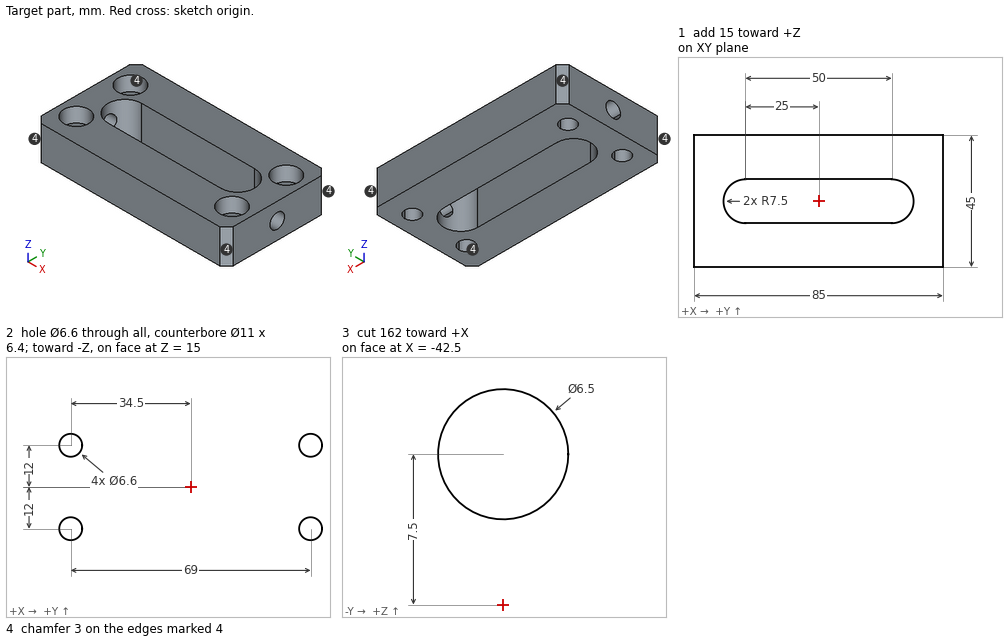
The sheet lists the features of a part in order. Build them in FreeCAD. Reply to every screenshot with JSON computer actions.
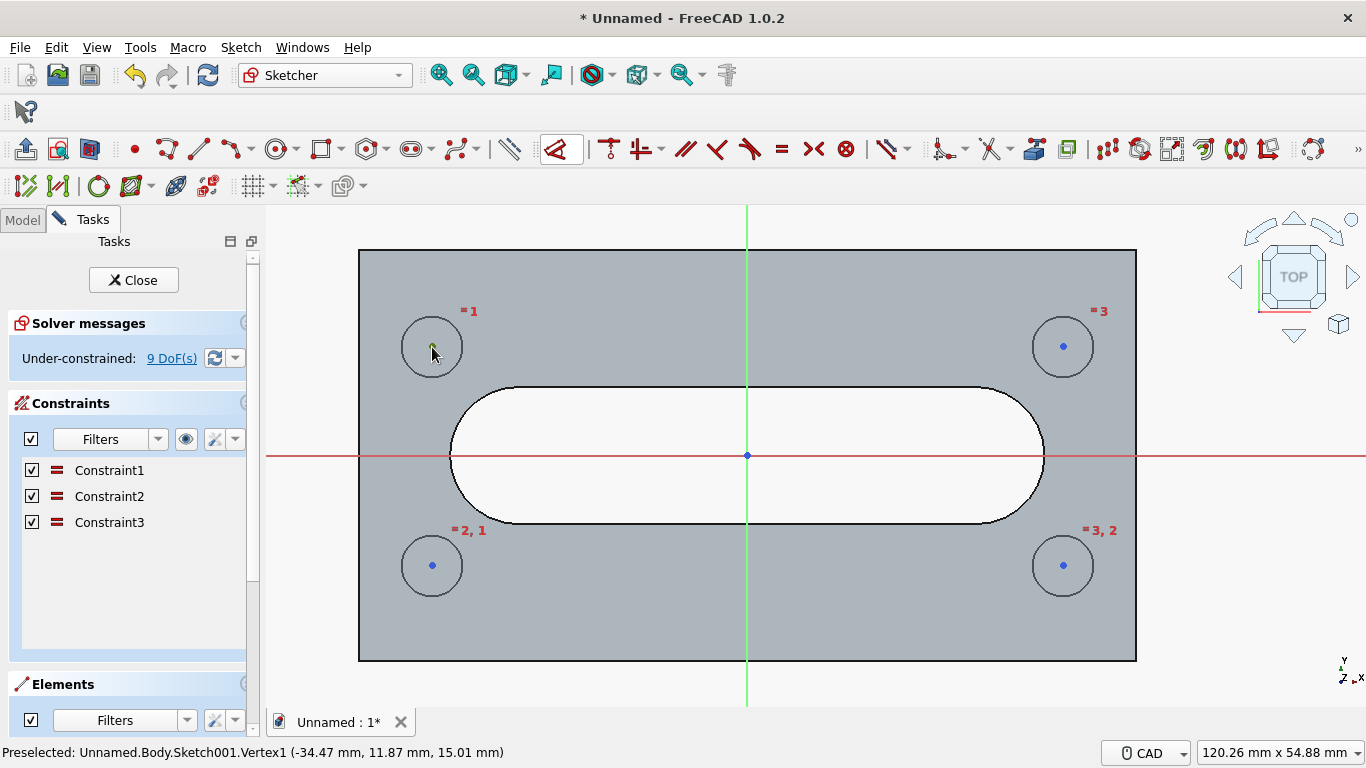
{"action": "left_click", "coordinate": [432, 566]}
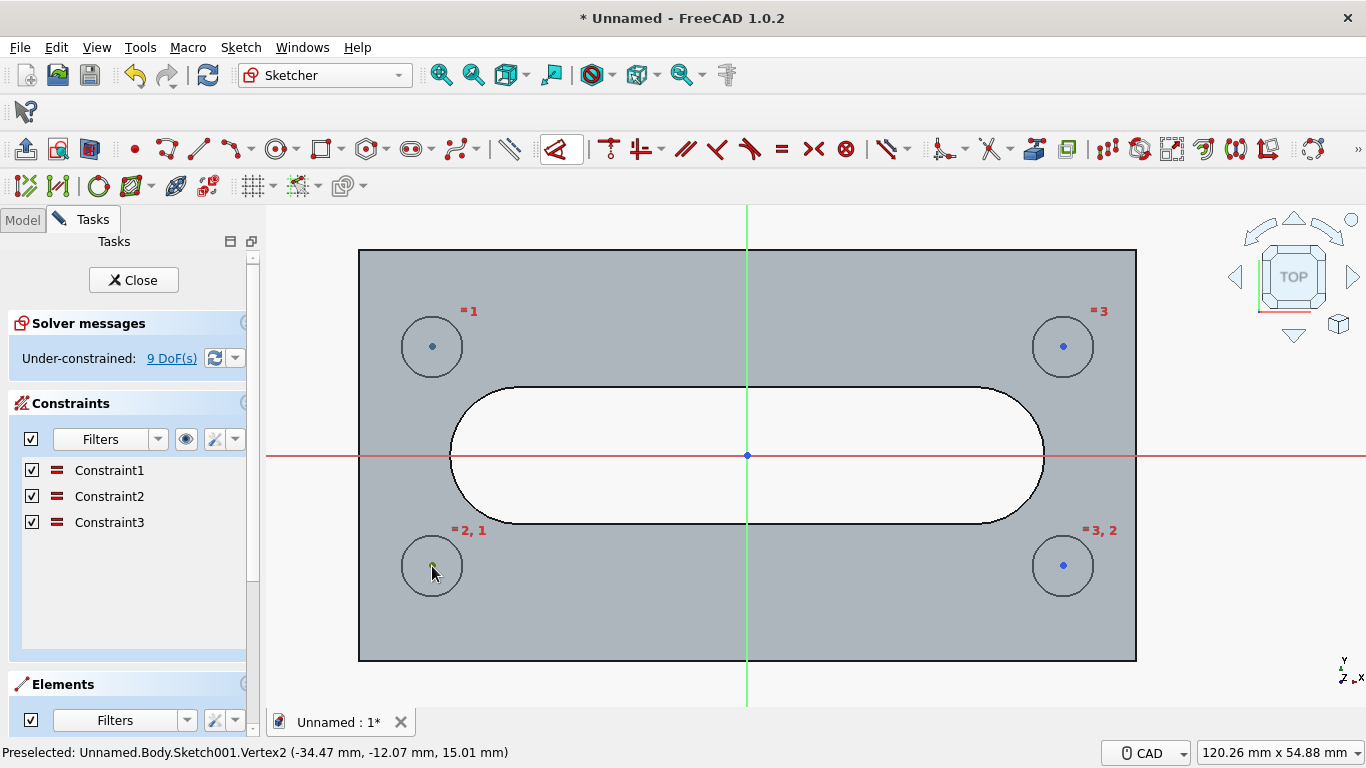
{"action": "left_click", "coordinate": [664, 150]}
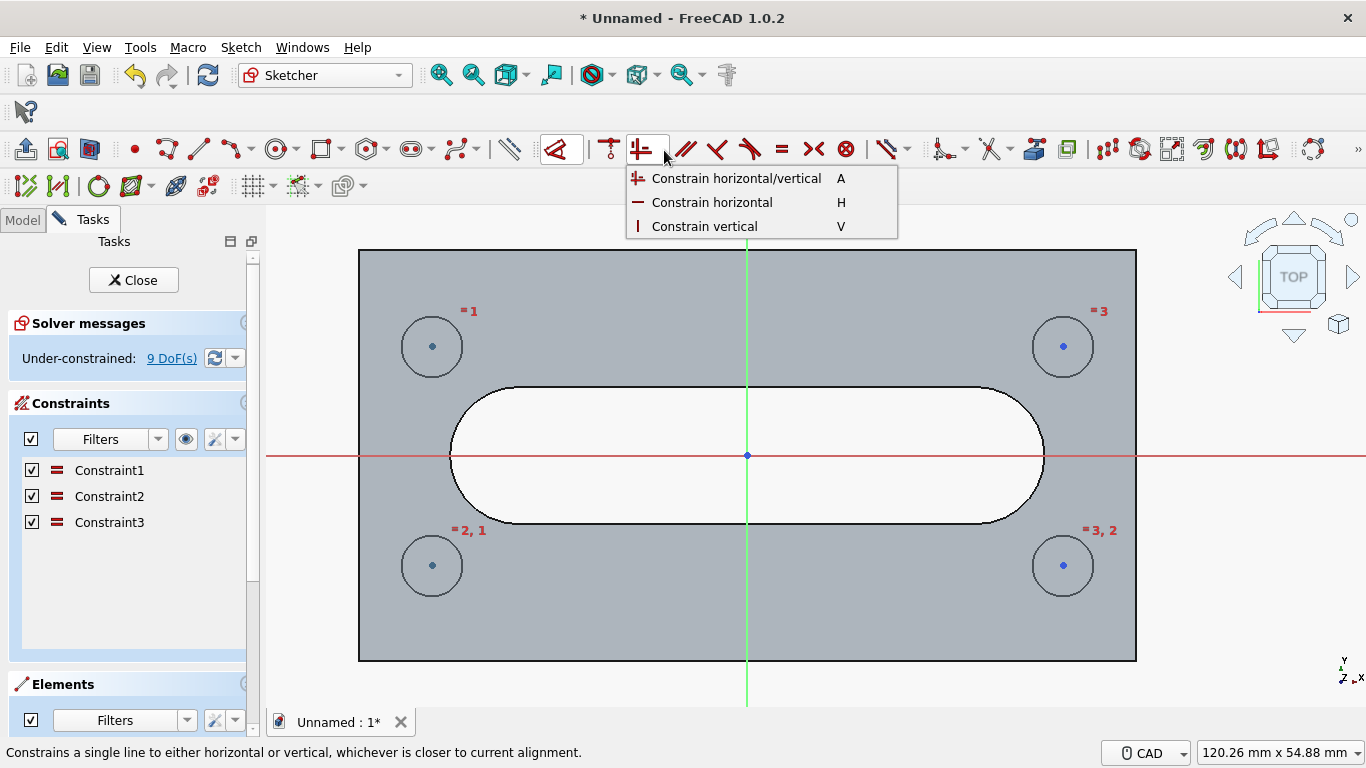
{"action": "left_click", "coordinate": [762, 226]}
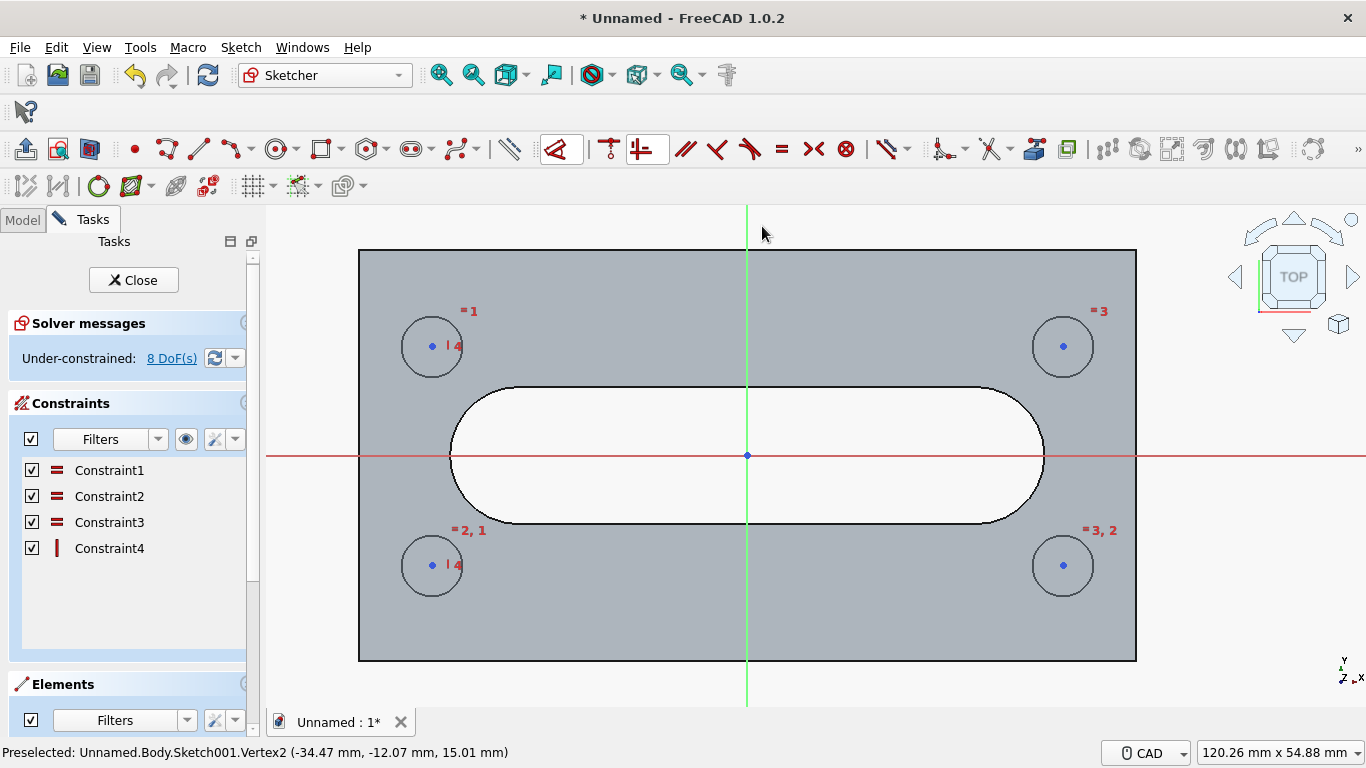
{"action": "left_click", "coordinate": [432, 566]}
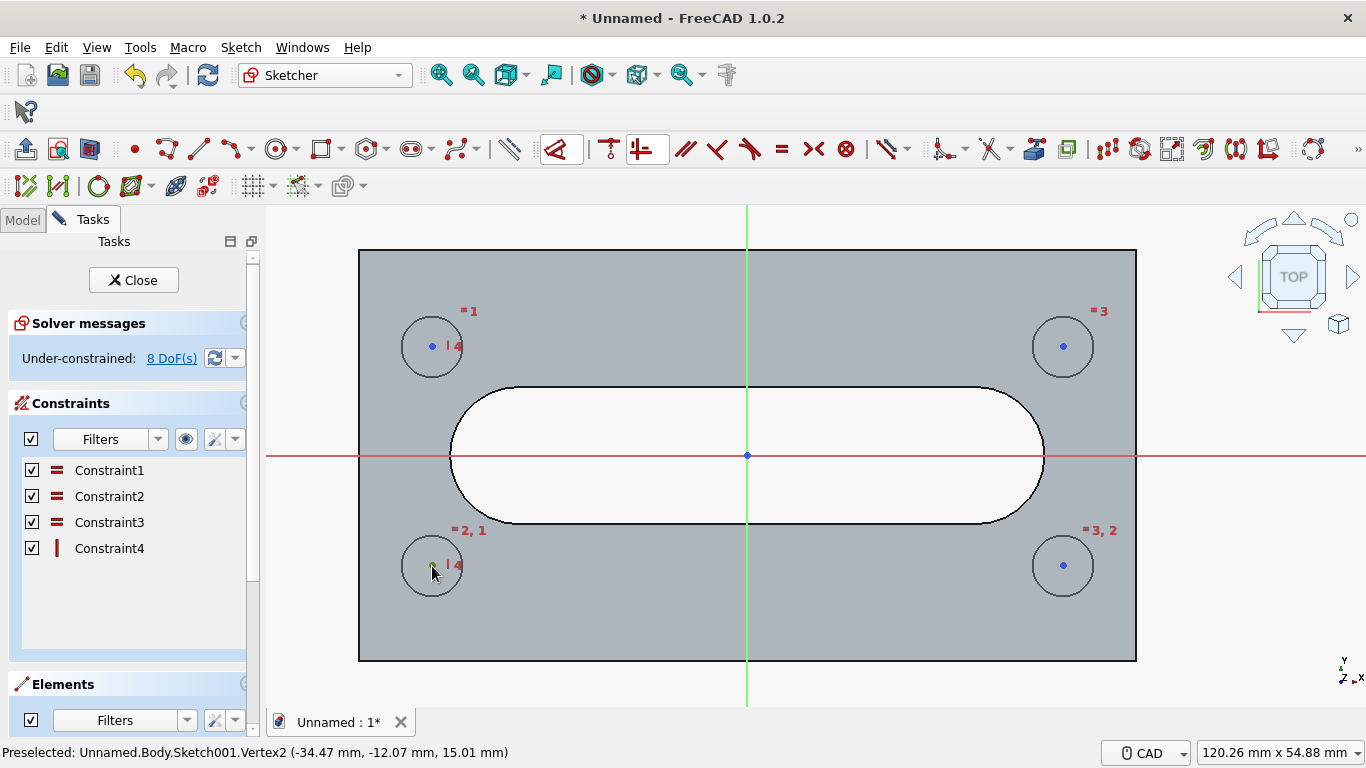
{"action": "left_click", "coordinate": [1063, 566]}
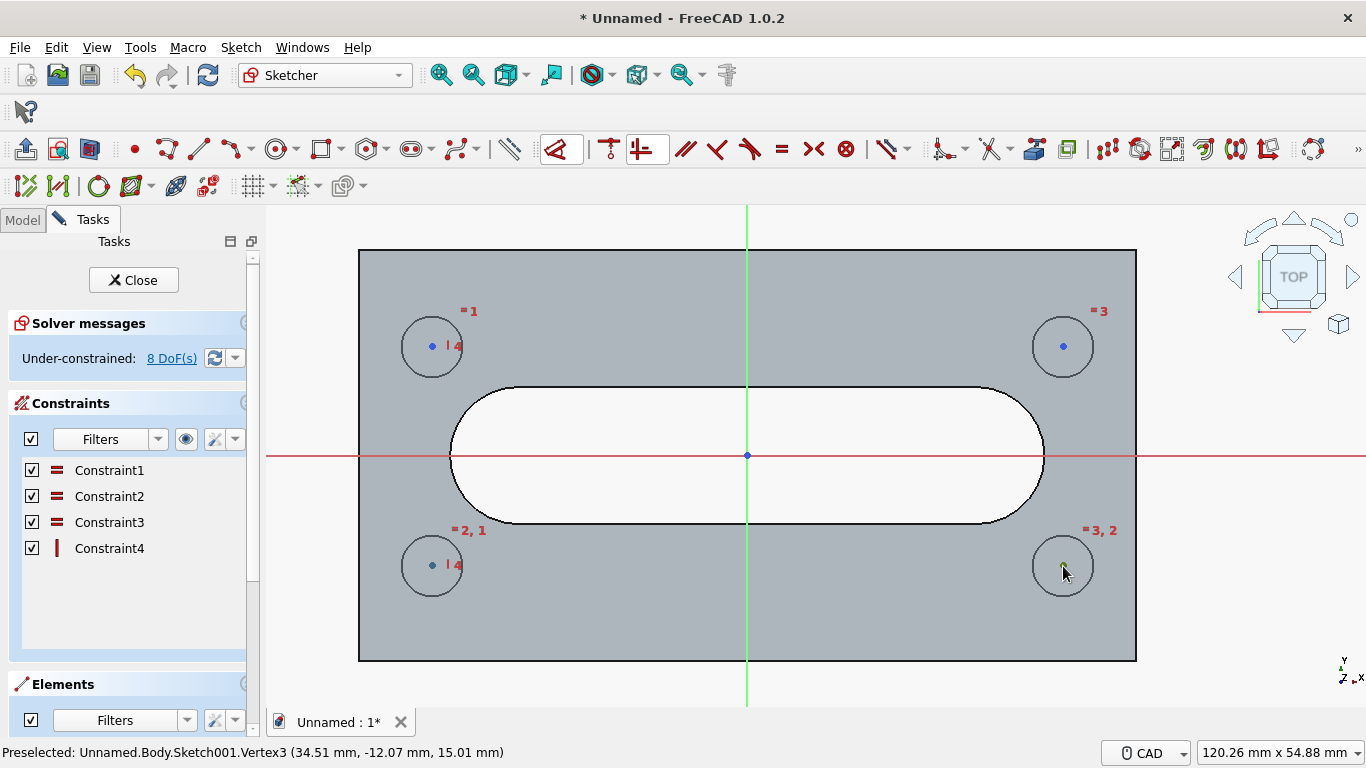
{"action": "left_click", "coordinate": [664, 150]}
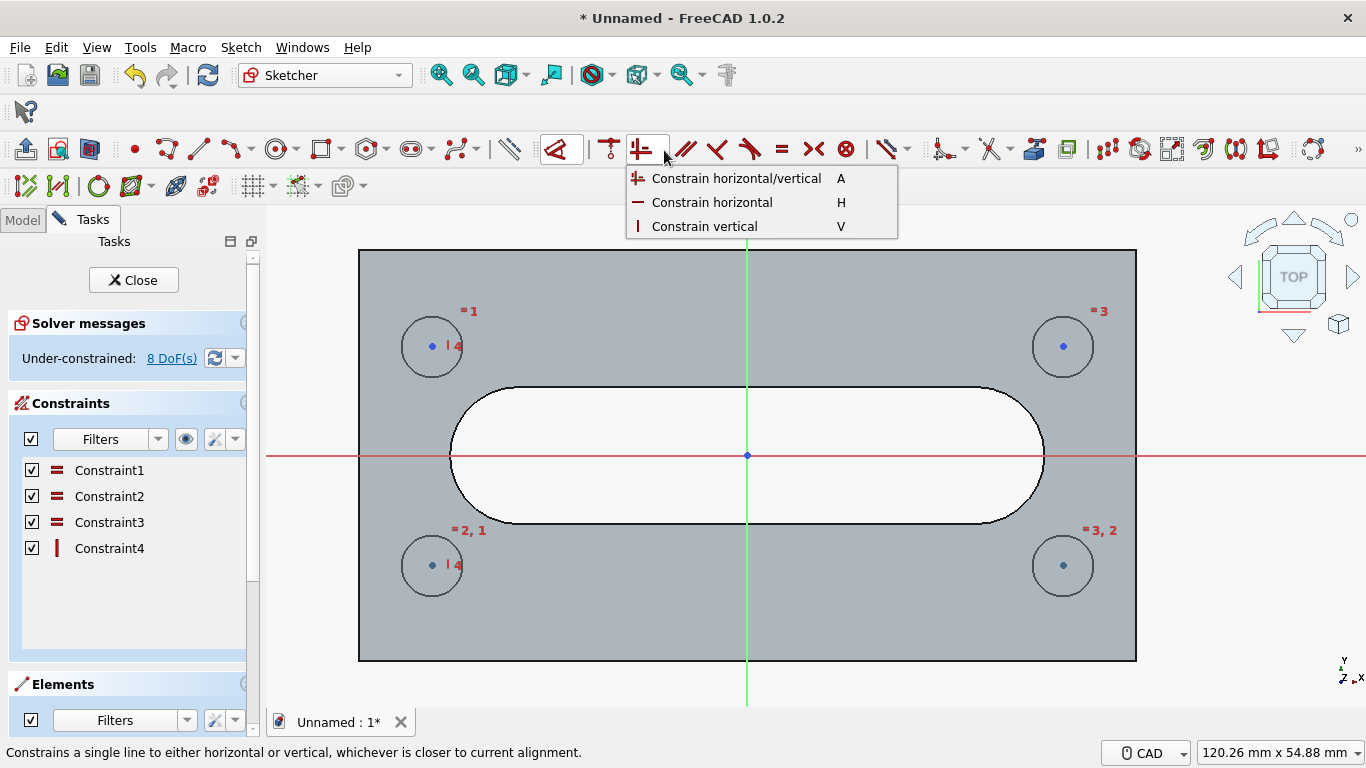
{"action": "left_click", "coordinate": [762, 202]}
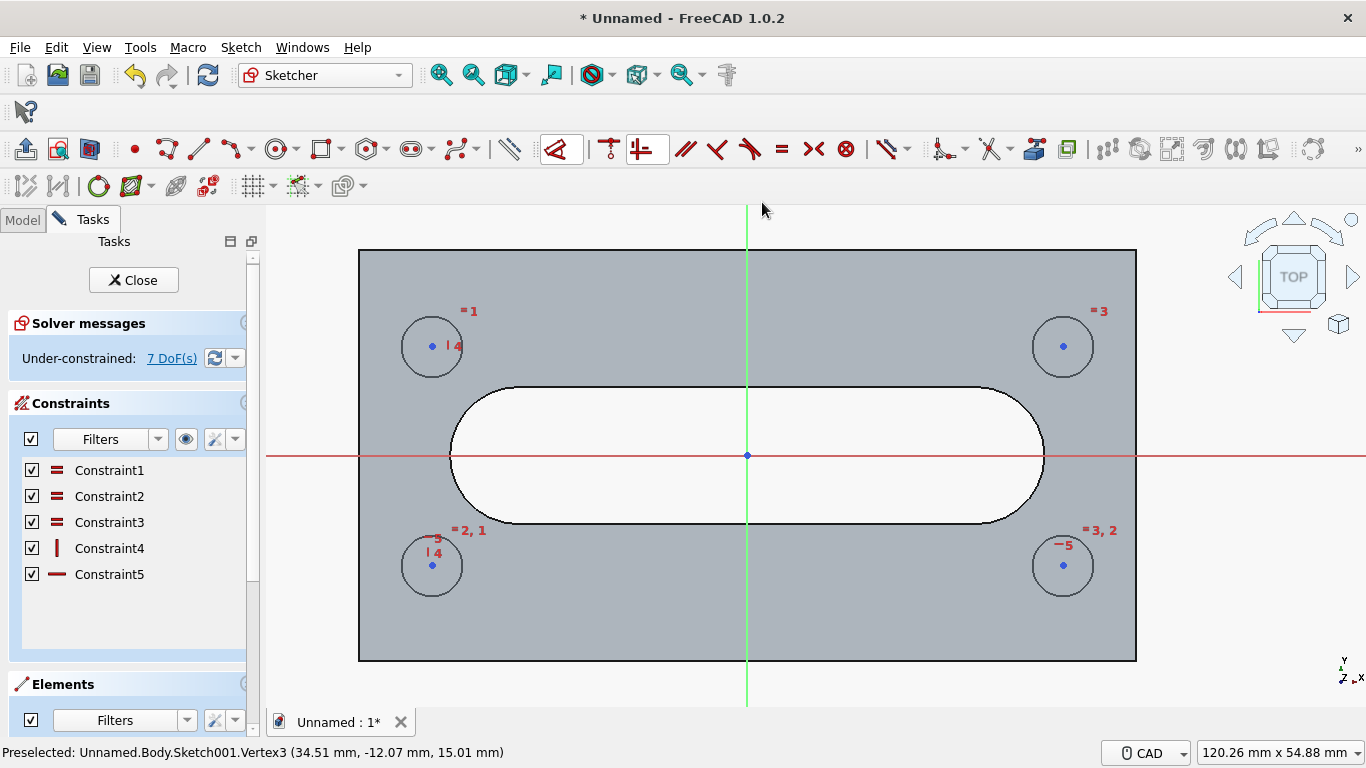
{"action": "left_click", "coordinate": [1063, 566]}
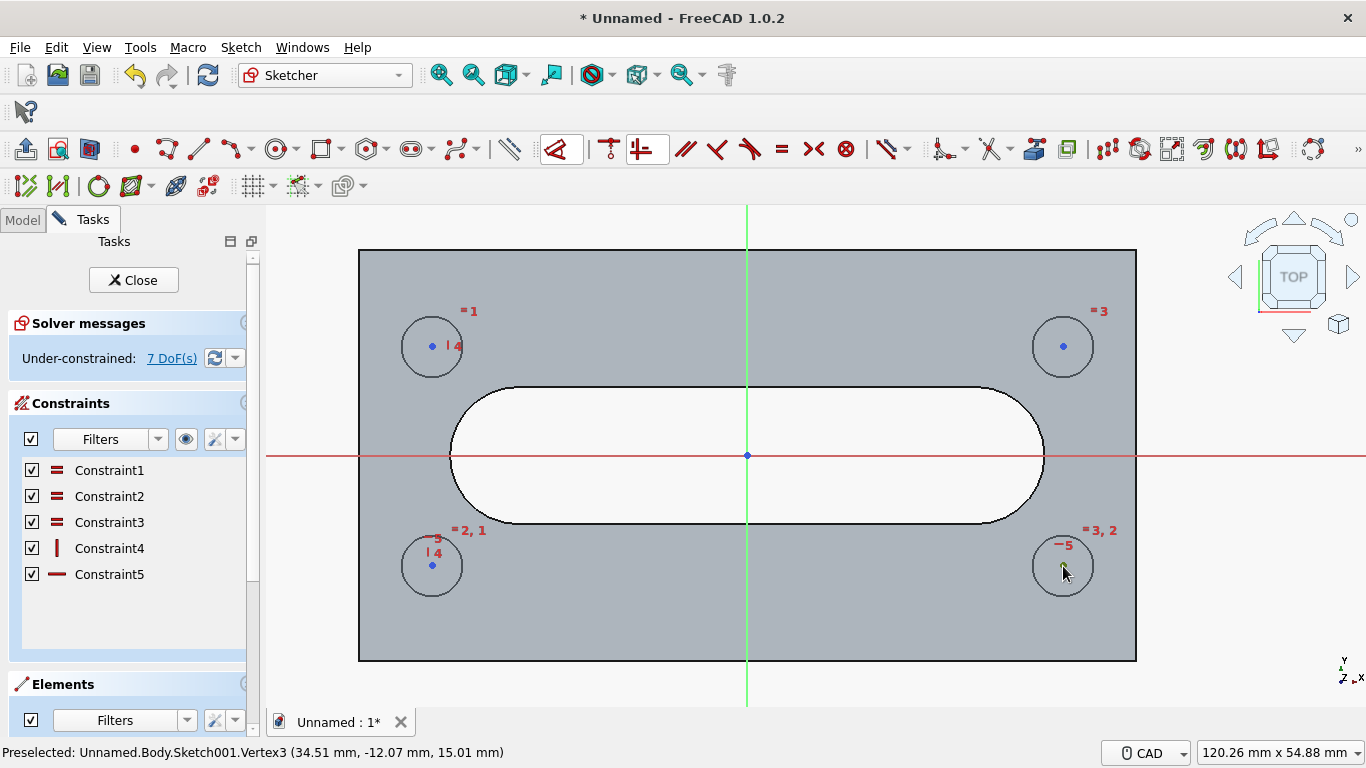
{"action": "left_click", "coordinate": [1063, 347]}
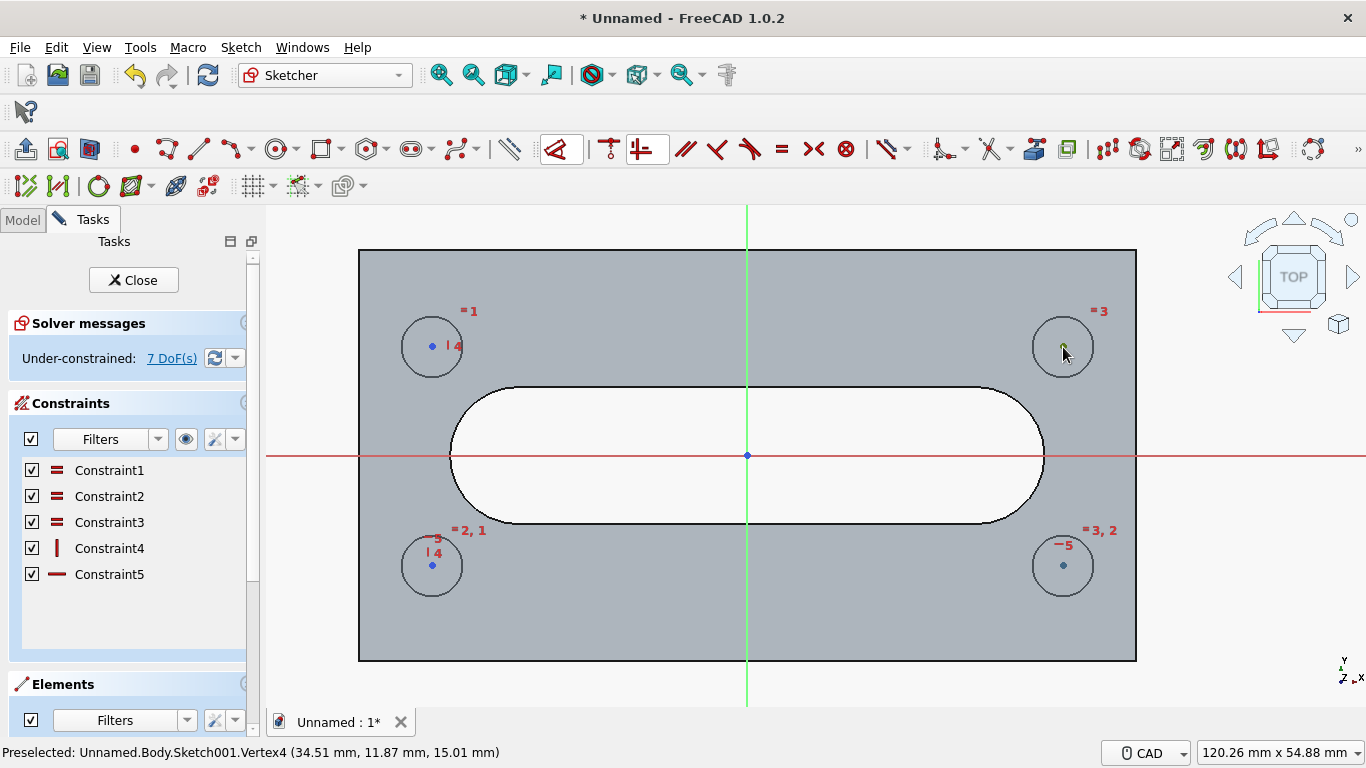
{"action": "left_click", "coordinate": [664, 150]}